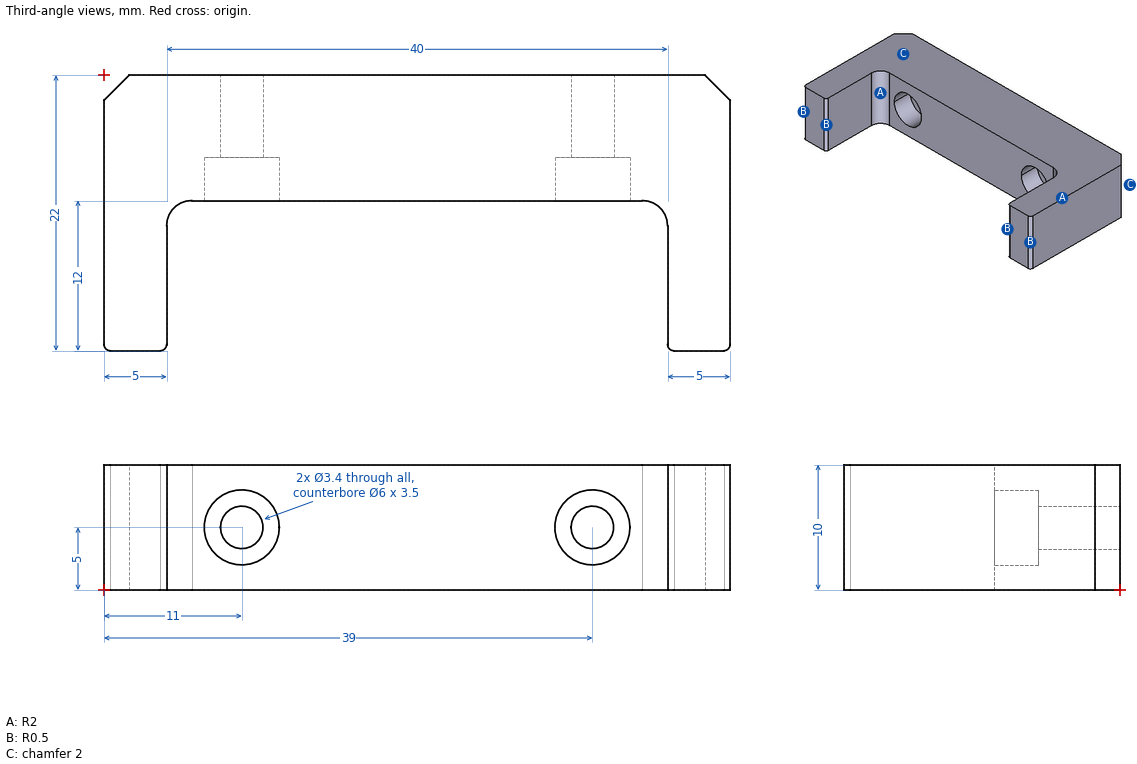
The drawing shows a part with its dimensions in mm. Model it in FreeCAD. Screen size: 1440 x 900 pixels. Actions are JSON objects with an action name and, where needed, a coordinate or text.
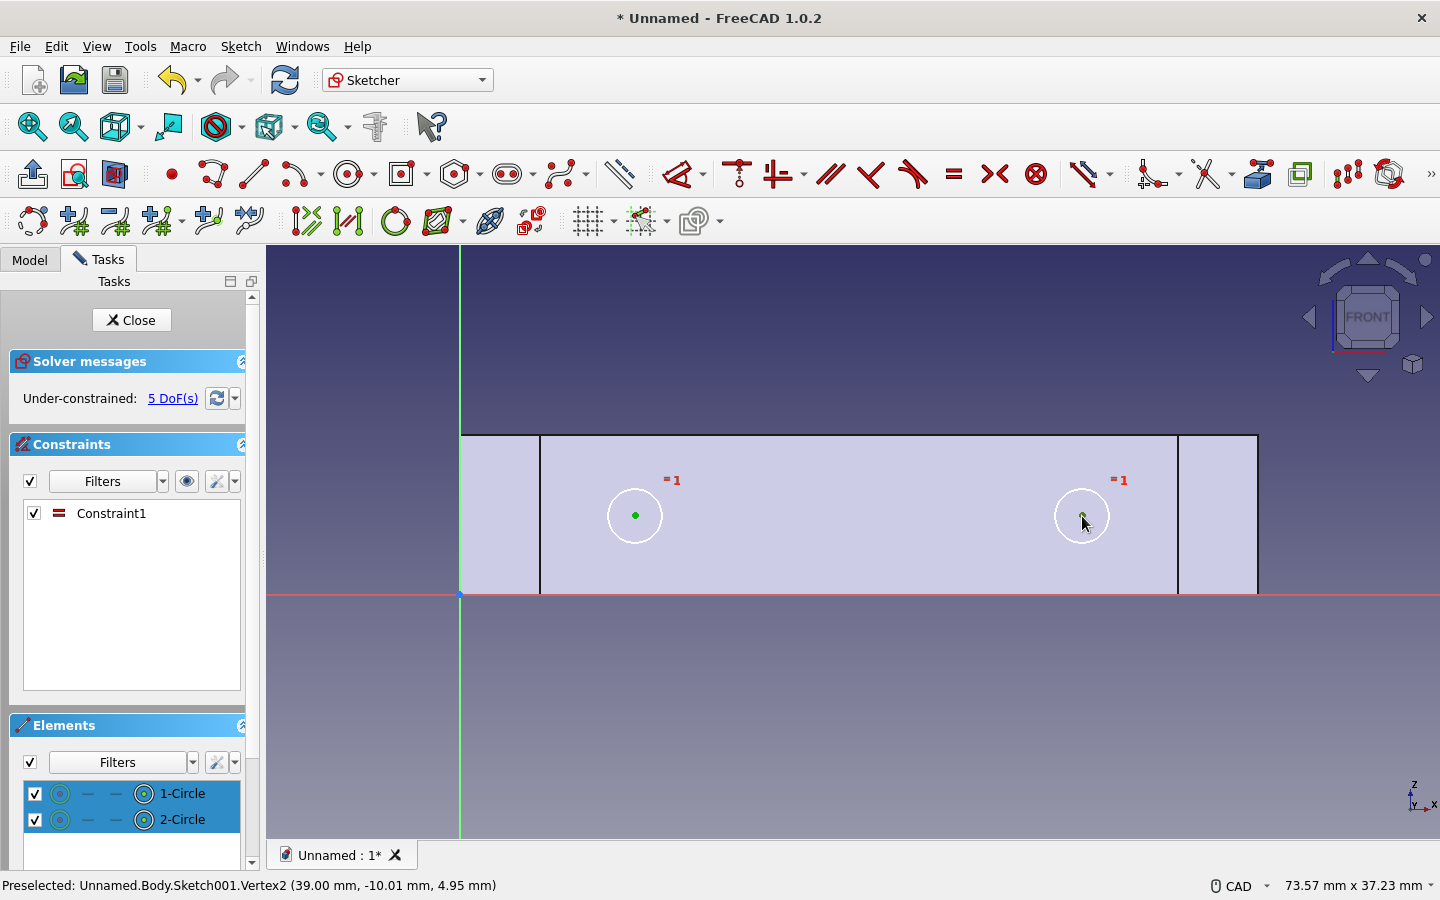
{"action": "left_click", "coordinate": [804, 174]}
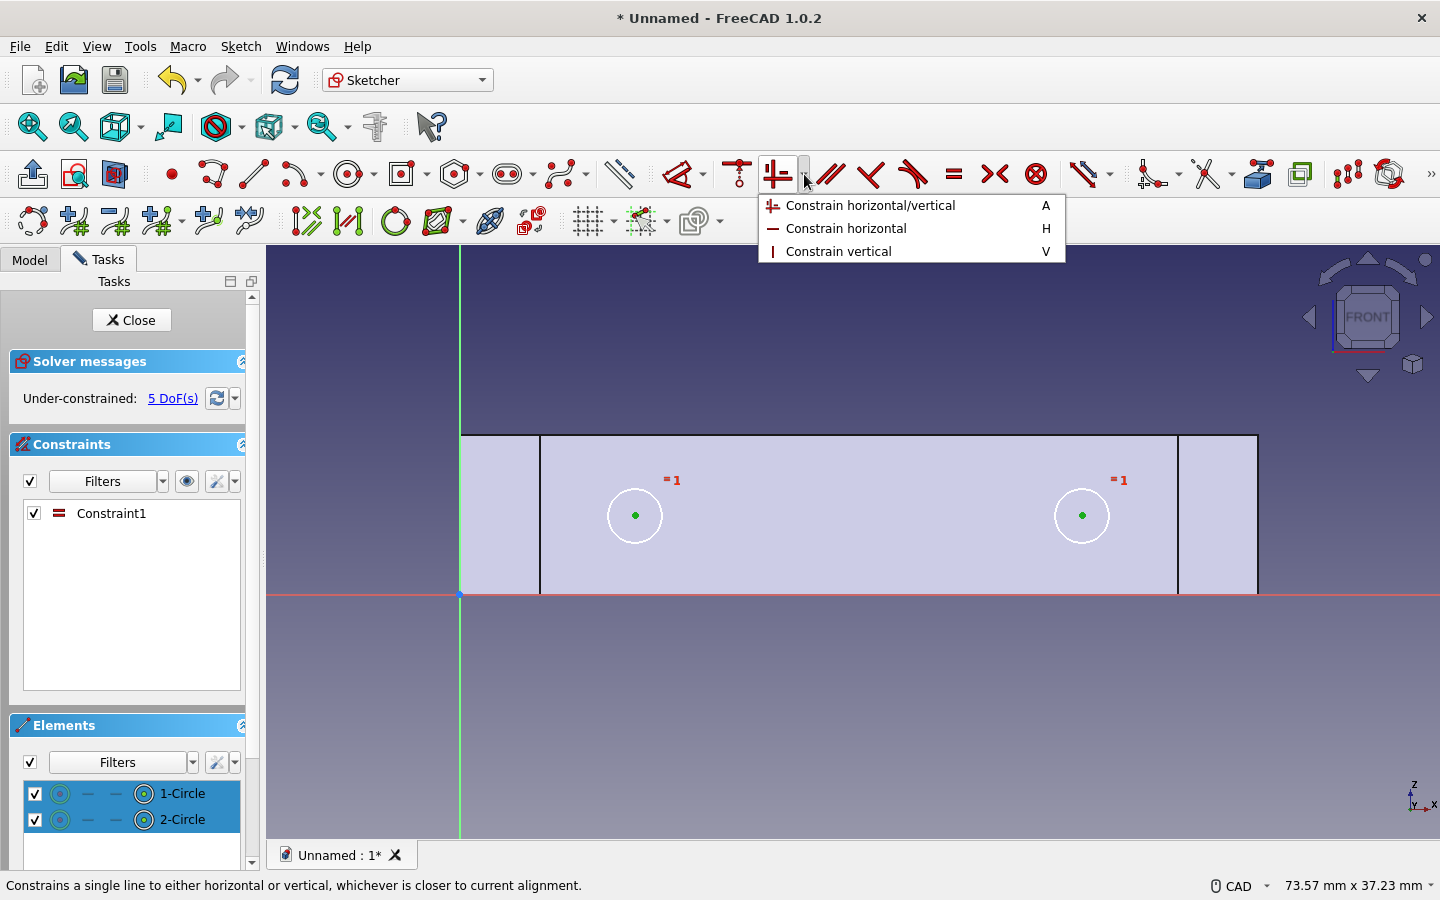
{"action": "left_click", "coordinate": [912, 228]}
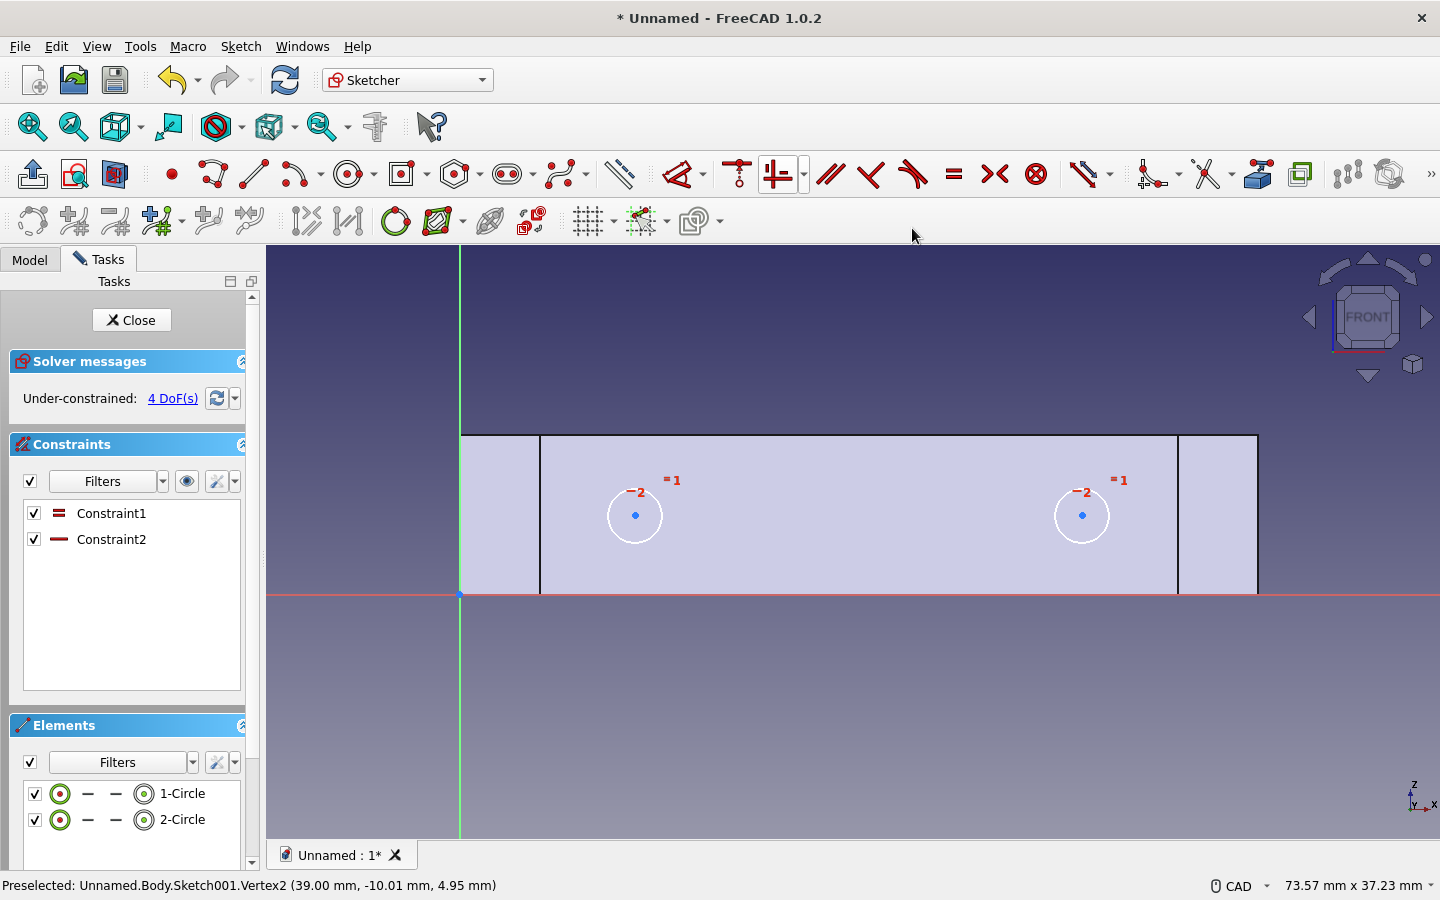
{"action": "left_click", "coordinate": [676, 174]}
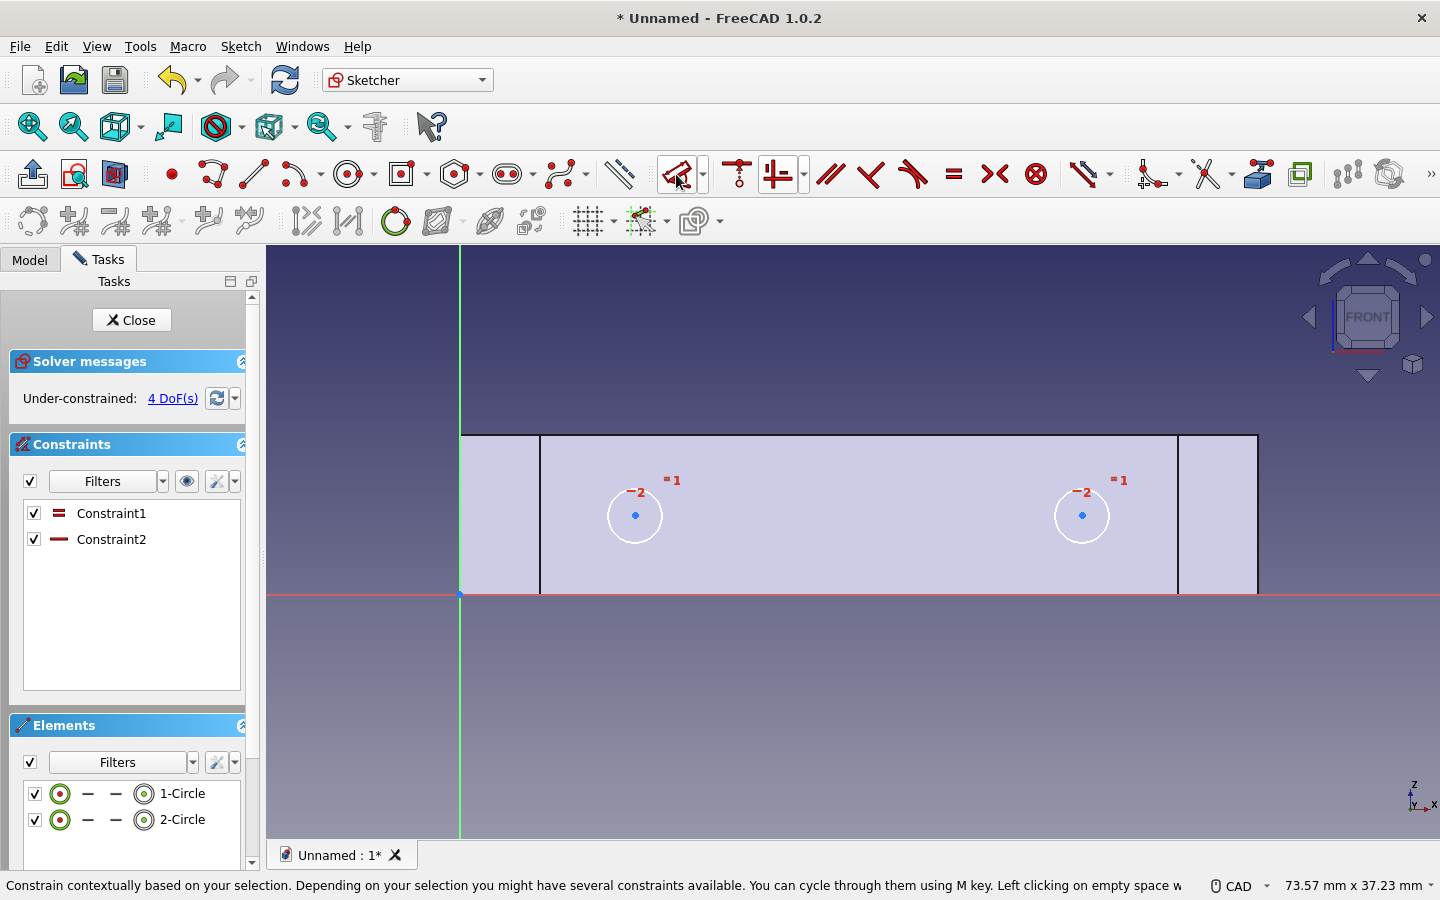
{"action": "left_click", "coordinate": [654, 497]}
{"action": "left_click", "coordinate": [677, 474]}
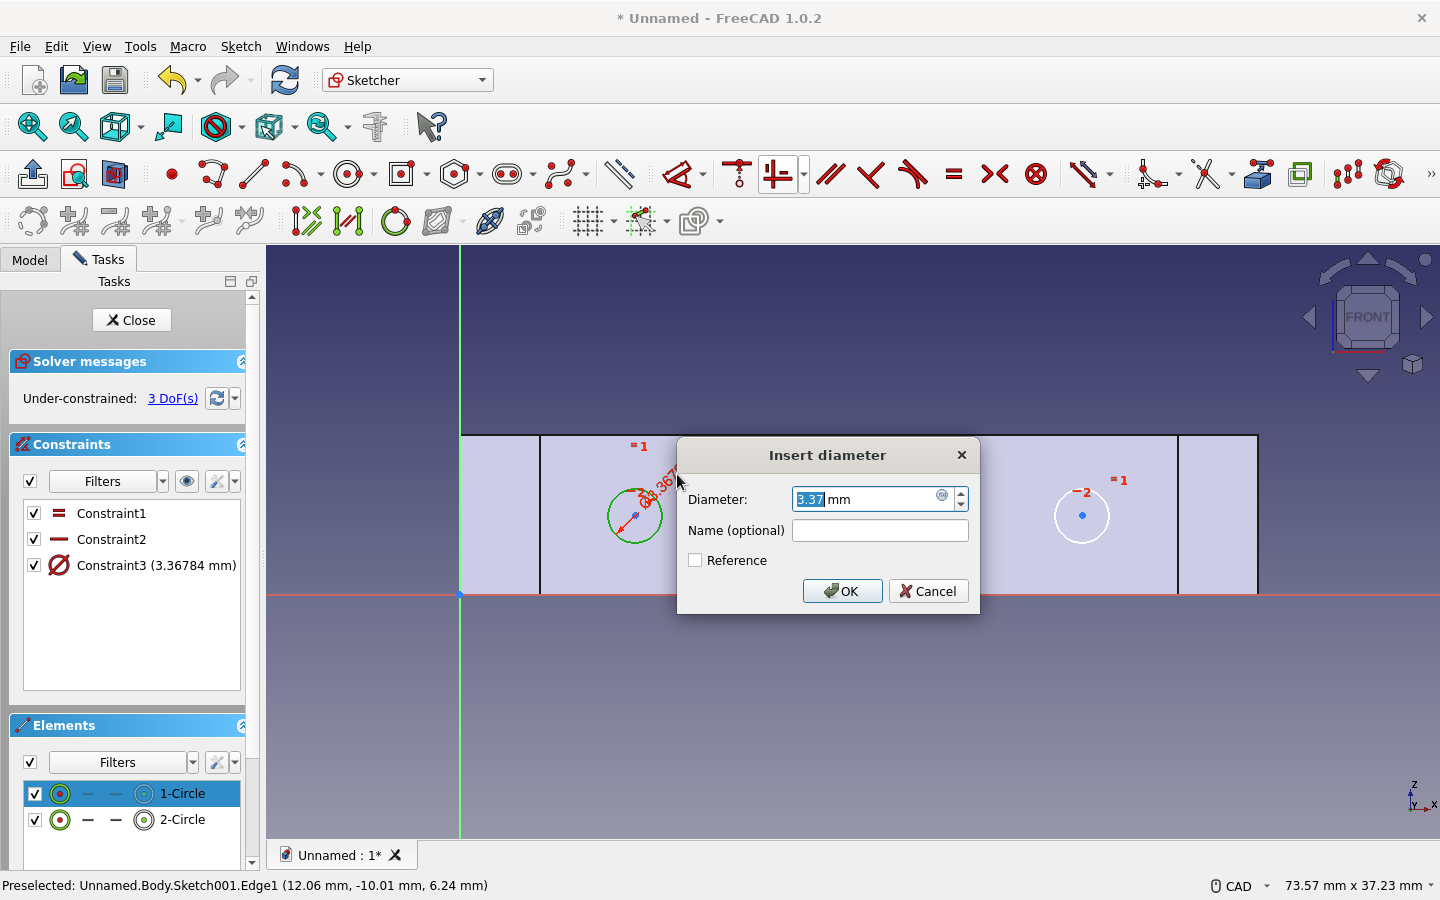
{"action": "type", "text": "3.4"}
{"action": "key", "text": "Return"}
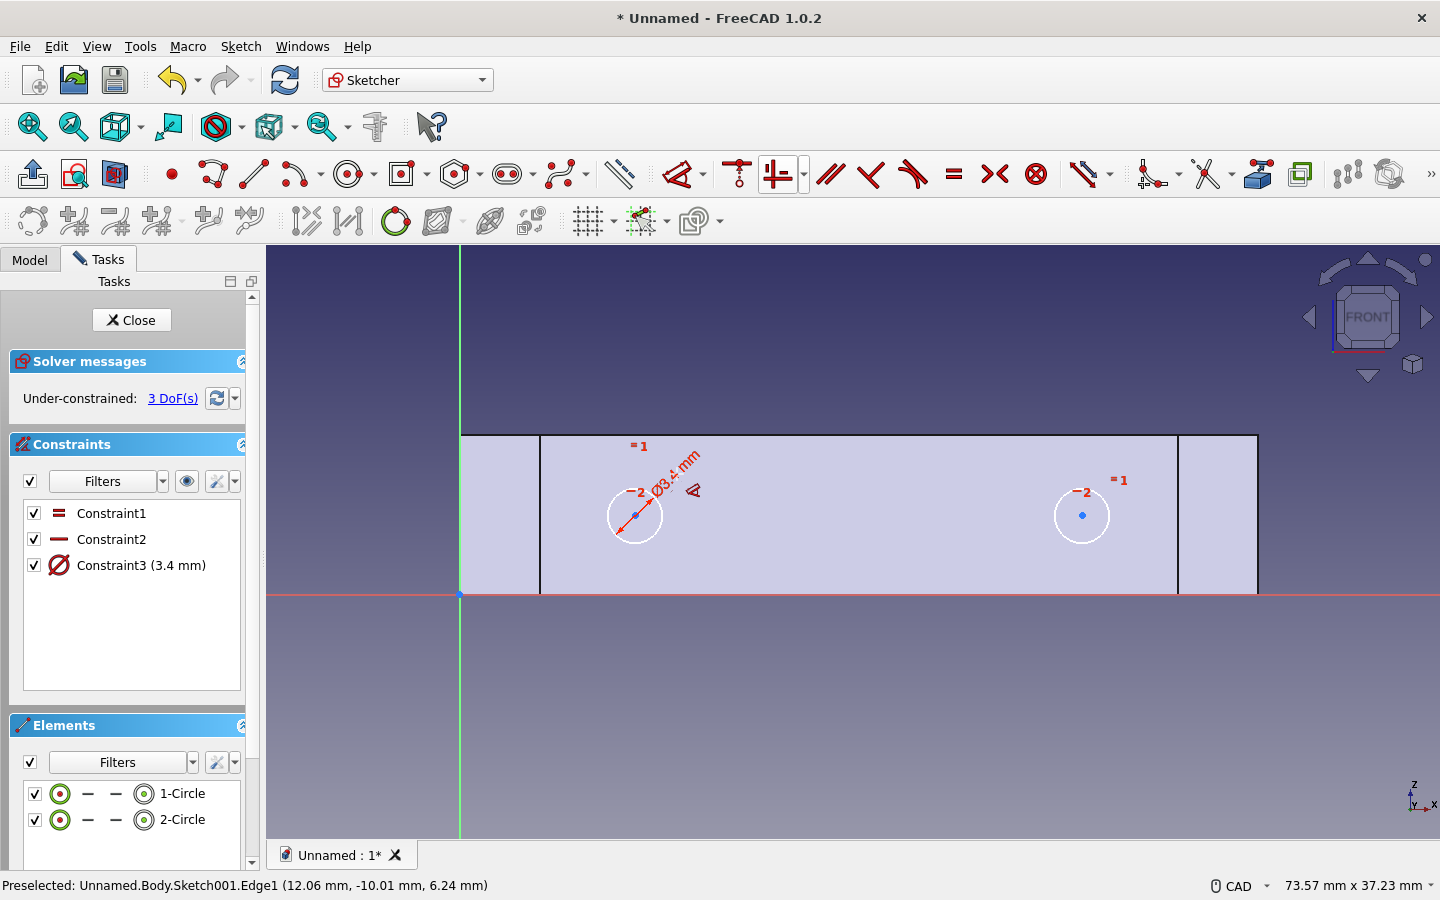
{"action": "left_click", "coordinate": [635, 516]}
{"action": "left_click", "coordinate": [426, 555]}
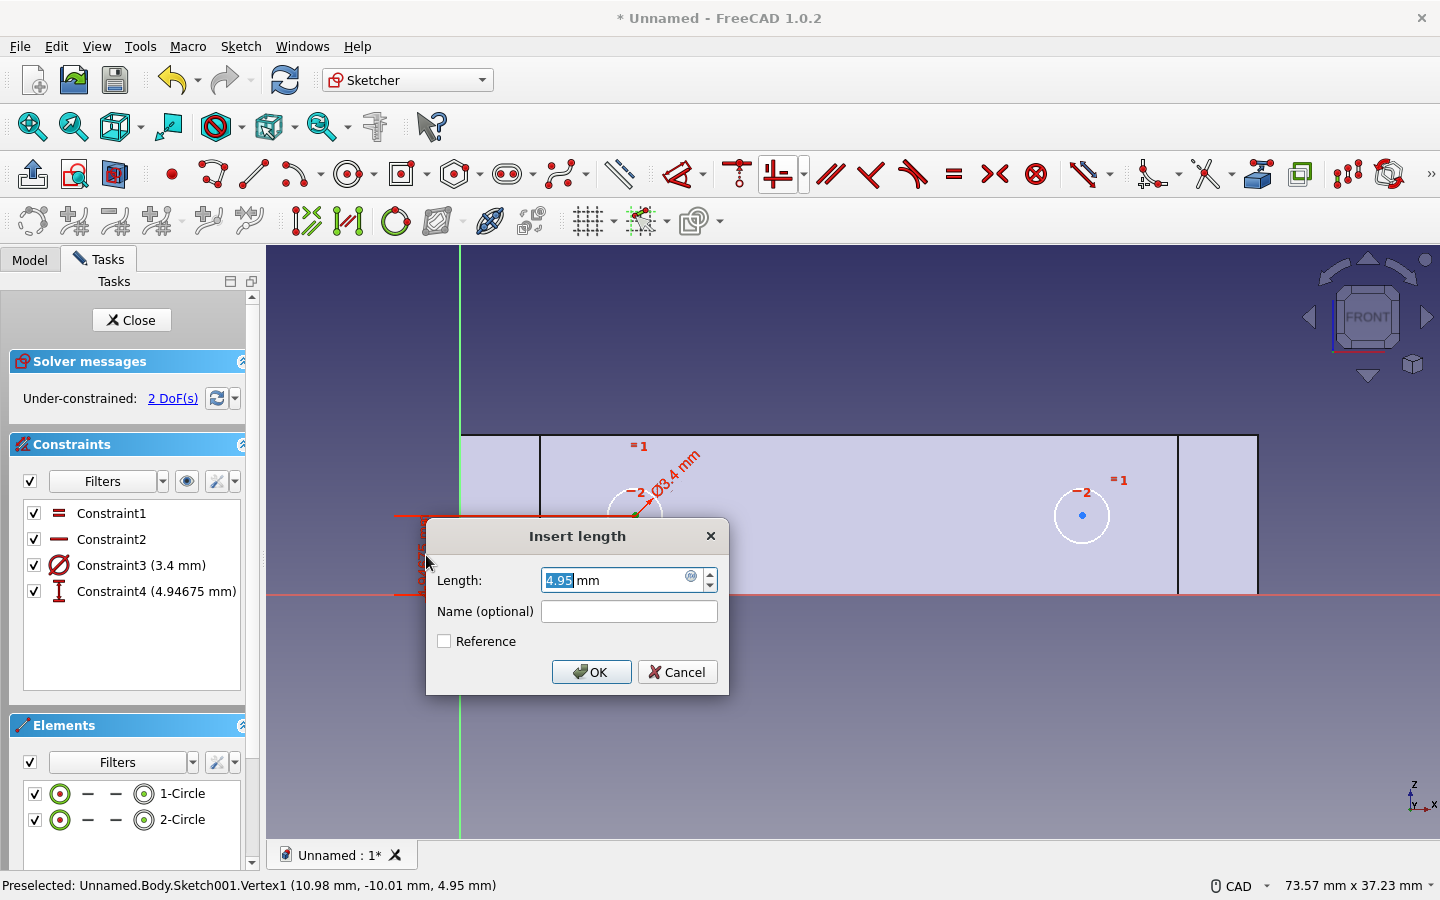
{"action": "type", "text": "5"}
{"action": "key", "text": "Return"}